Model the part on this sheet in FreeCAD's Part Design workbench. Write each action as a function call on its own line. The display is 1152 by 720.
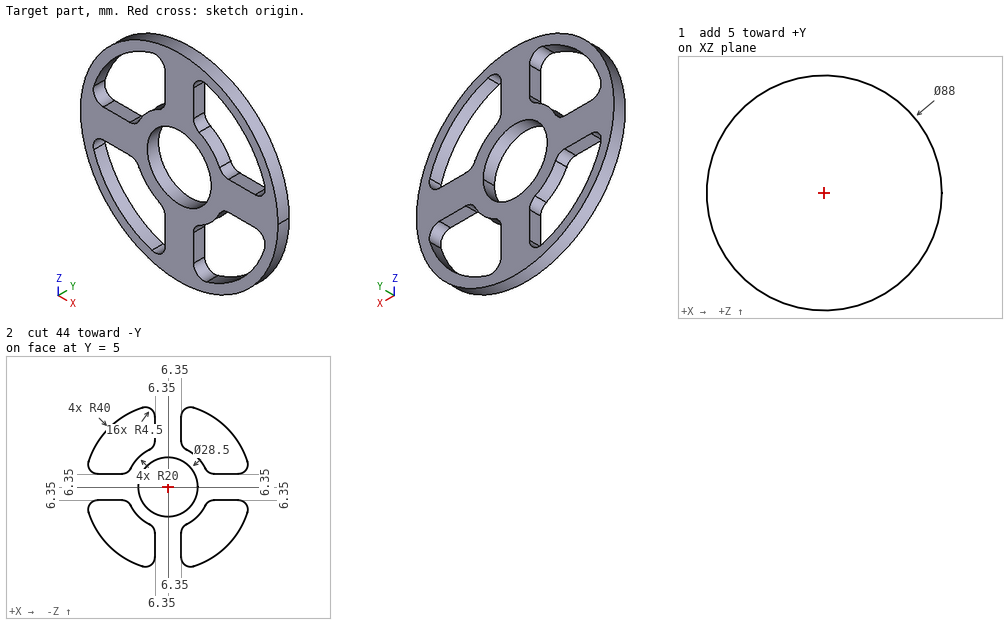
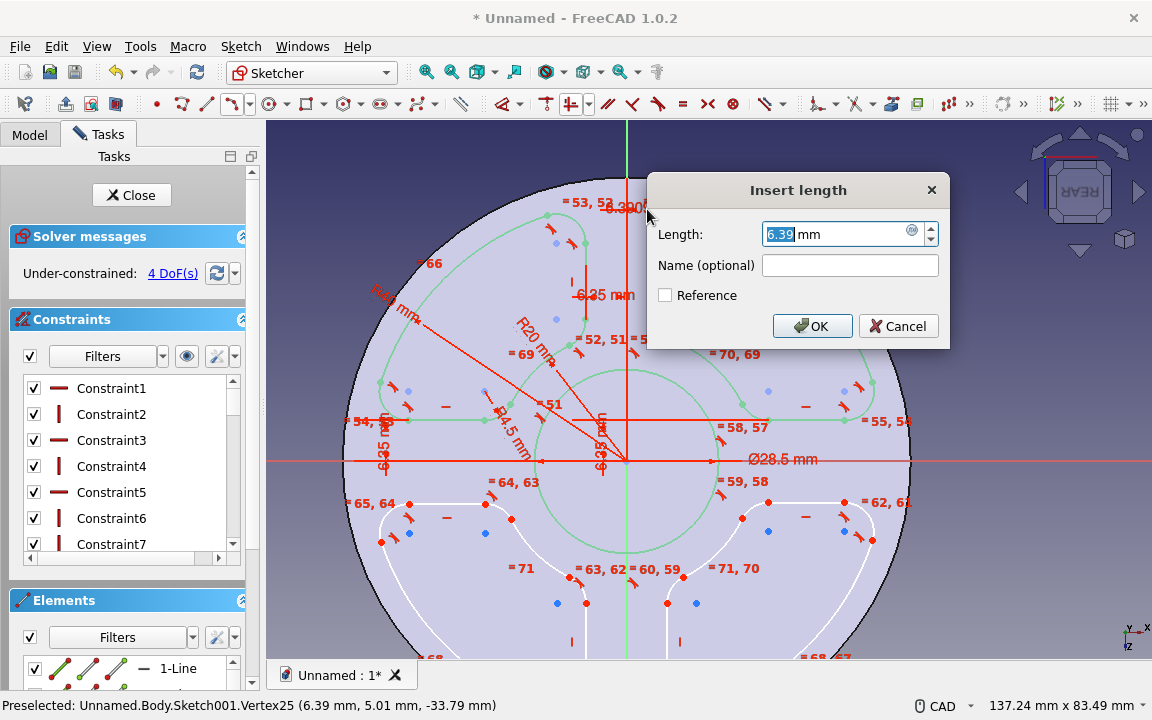
text(6.35)
key(Return)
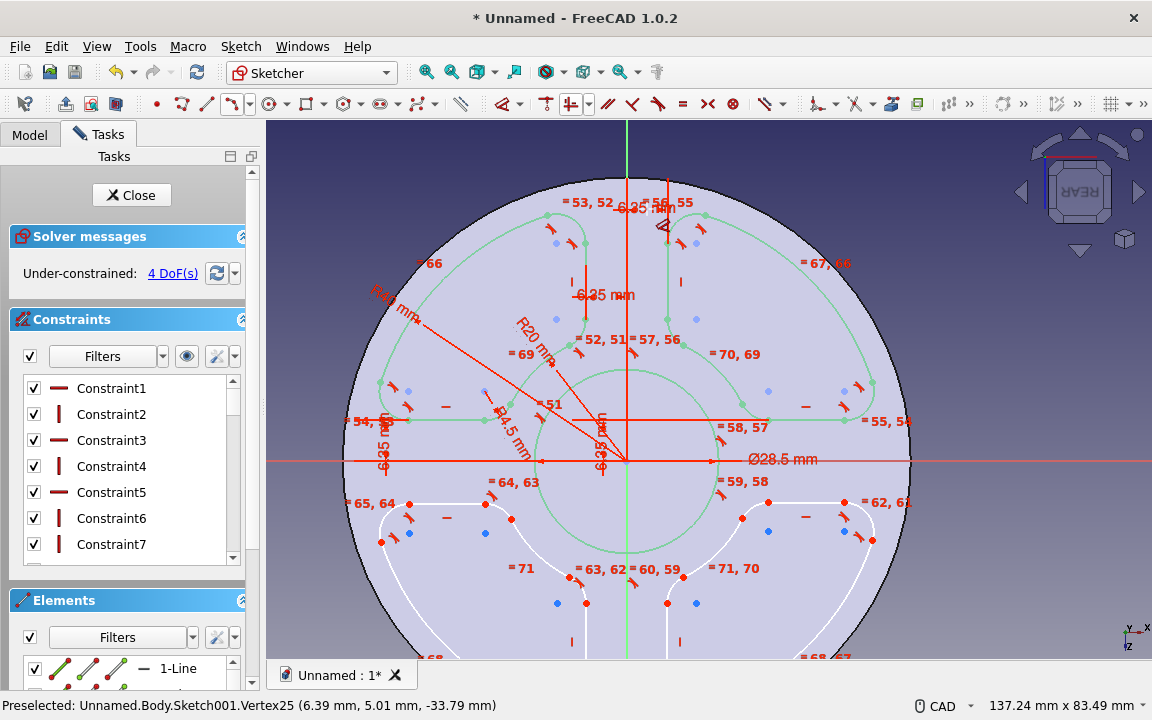
click(845, 503)
click(879, 482)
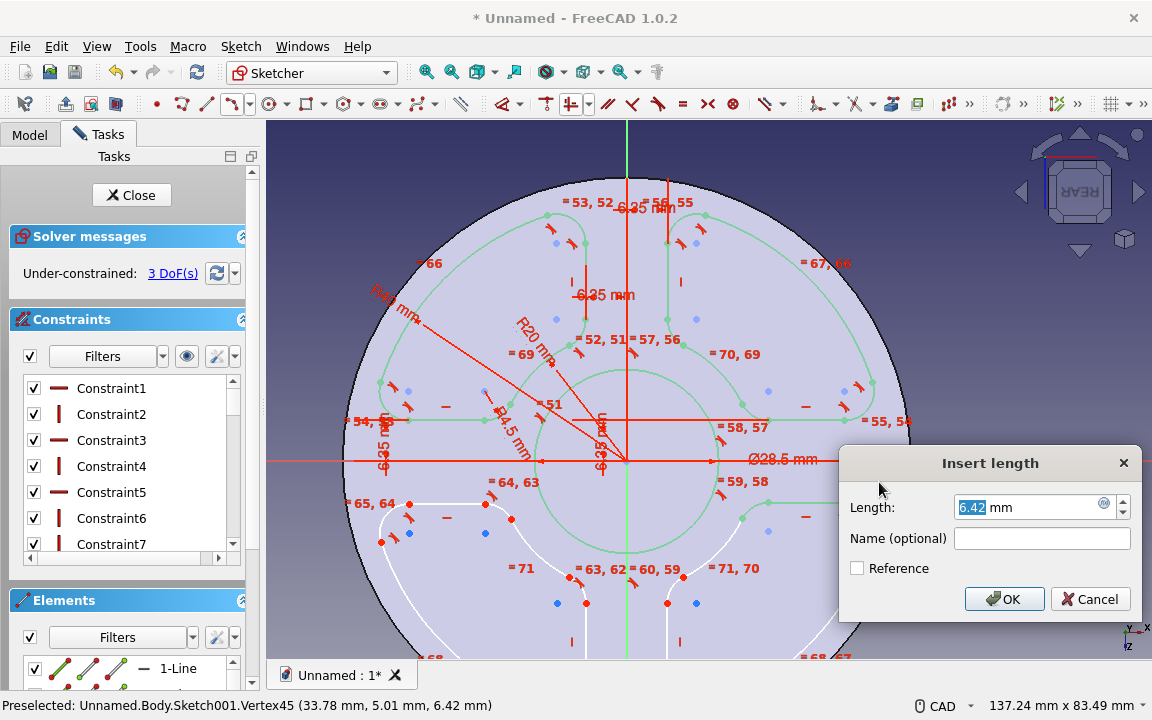
text(6.35)
key(Return)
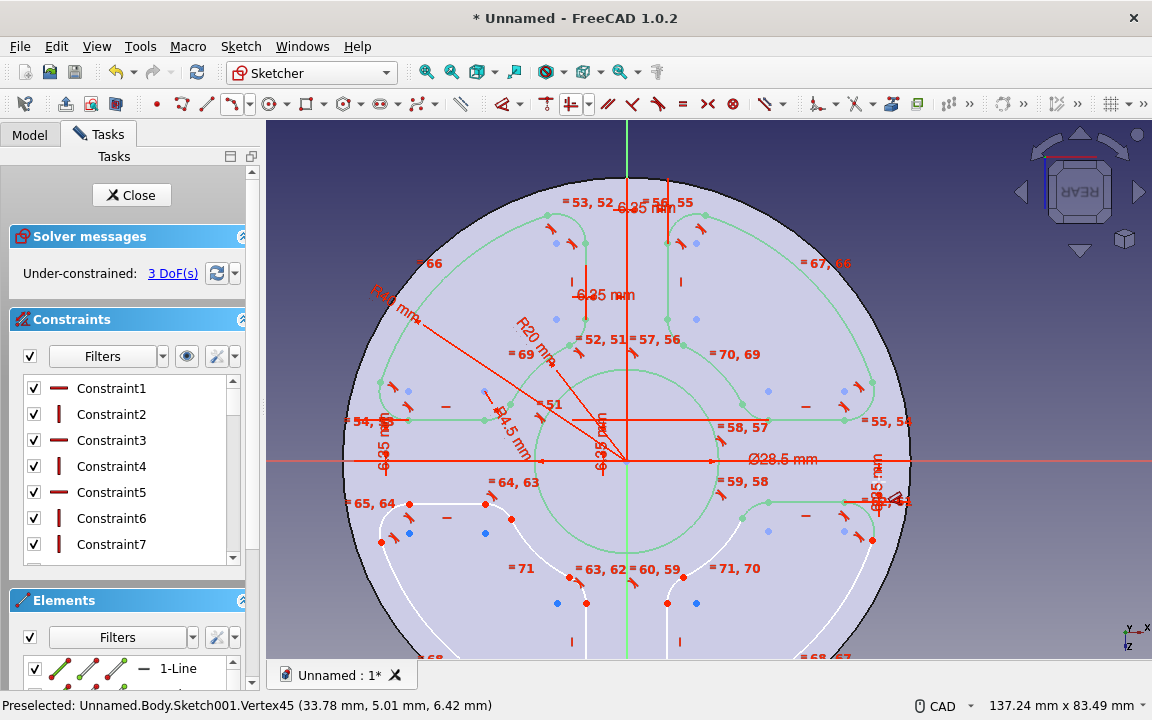
click(667, 604)
click(647, 403)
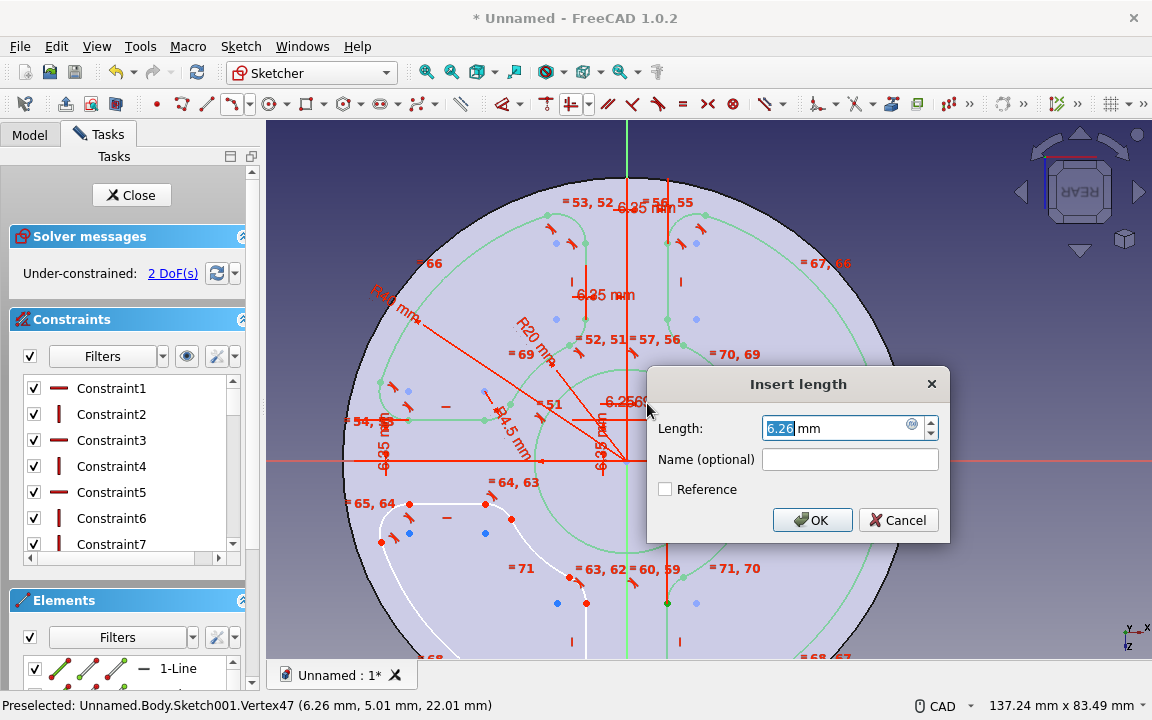
text(6.35)
key(Return)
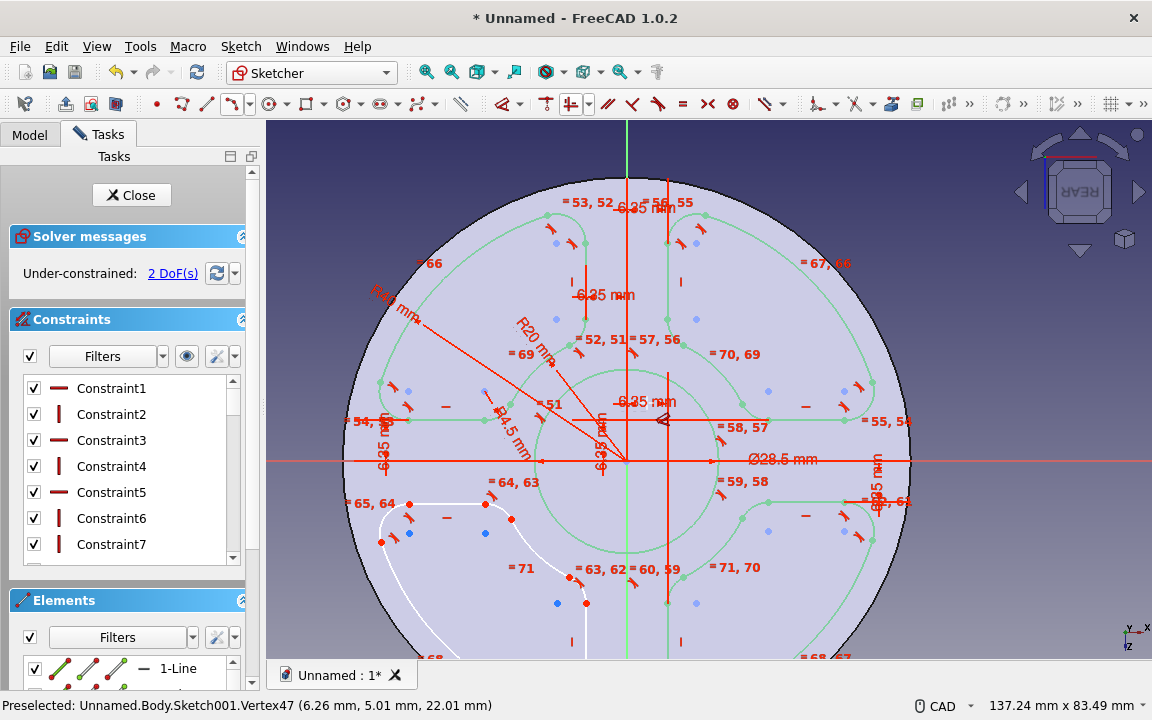
scroll(669, 243, down, 2)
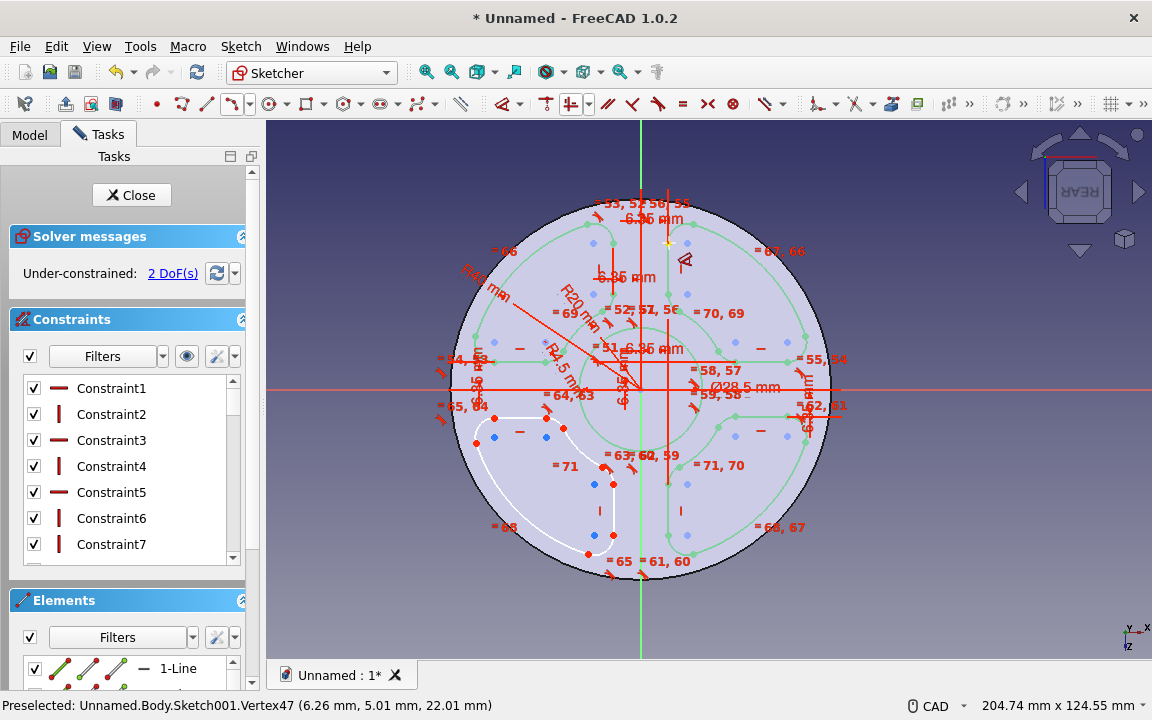
scroll(614, 536, up, 2)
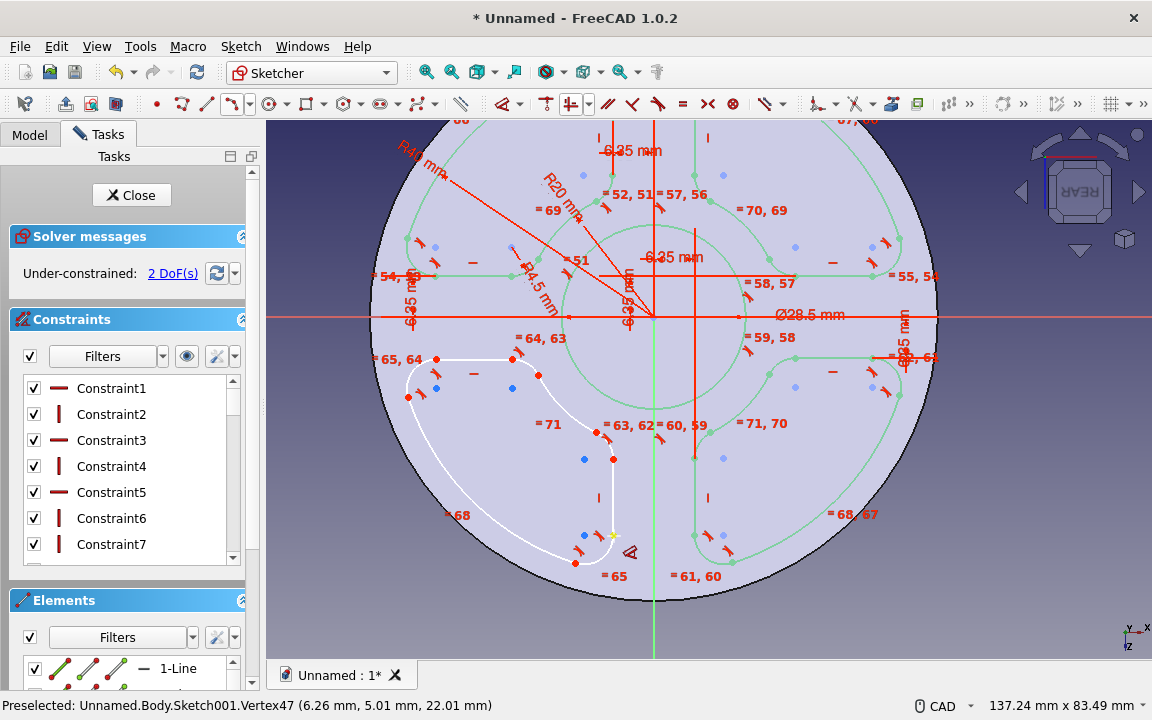
click(613, 535)
click(633, 569)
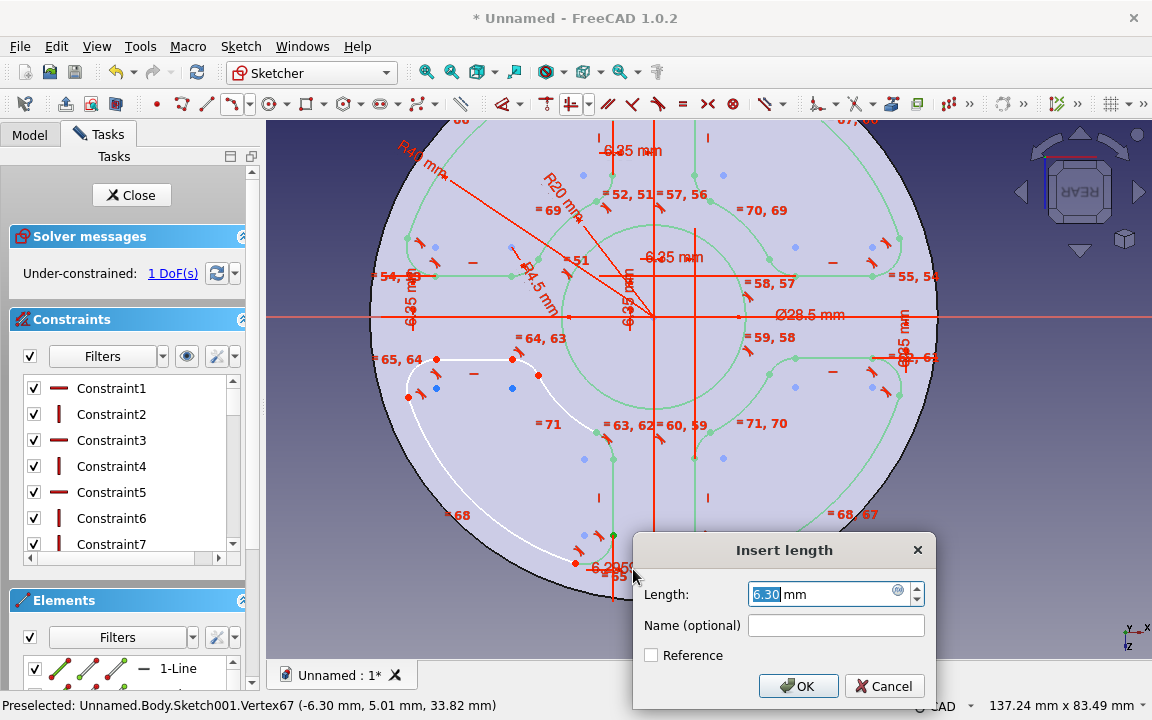
text(6.35)
key(Return)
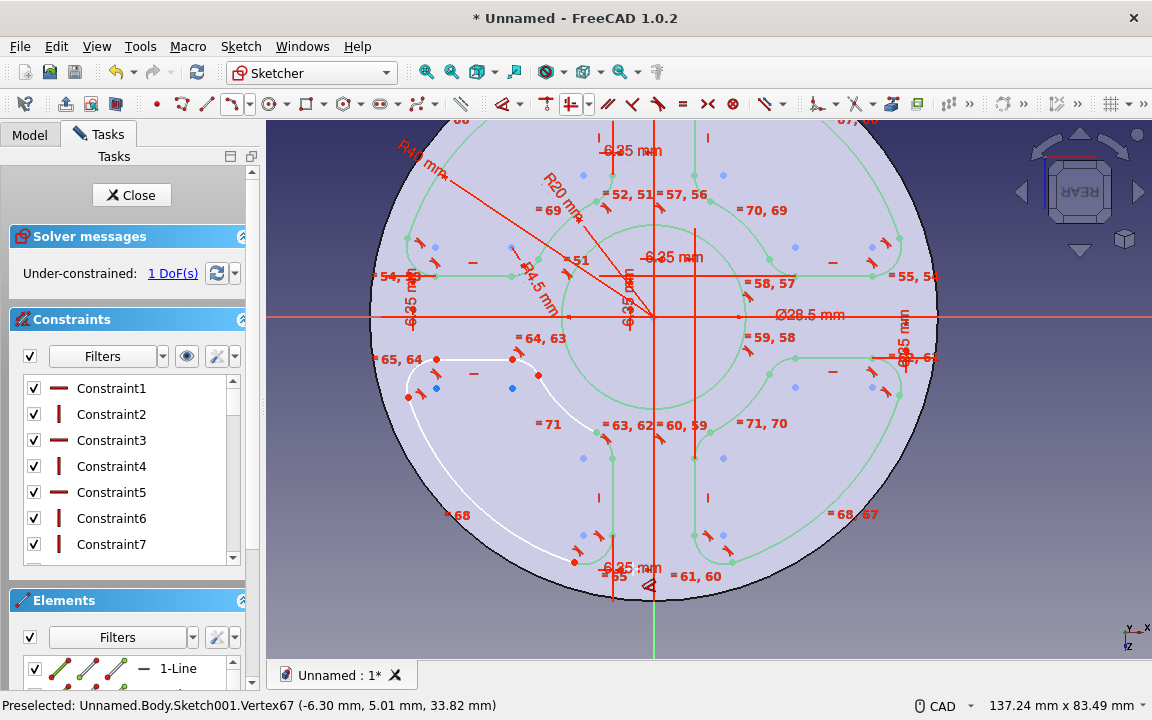
click(513, 360)
click(479, 338)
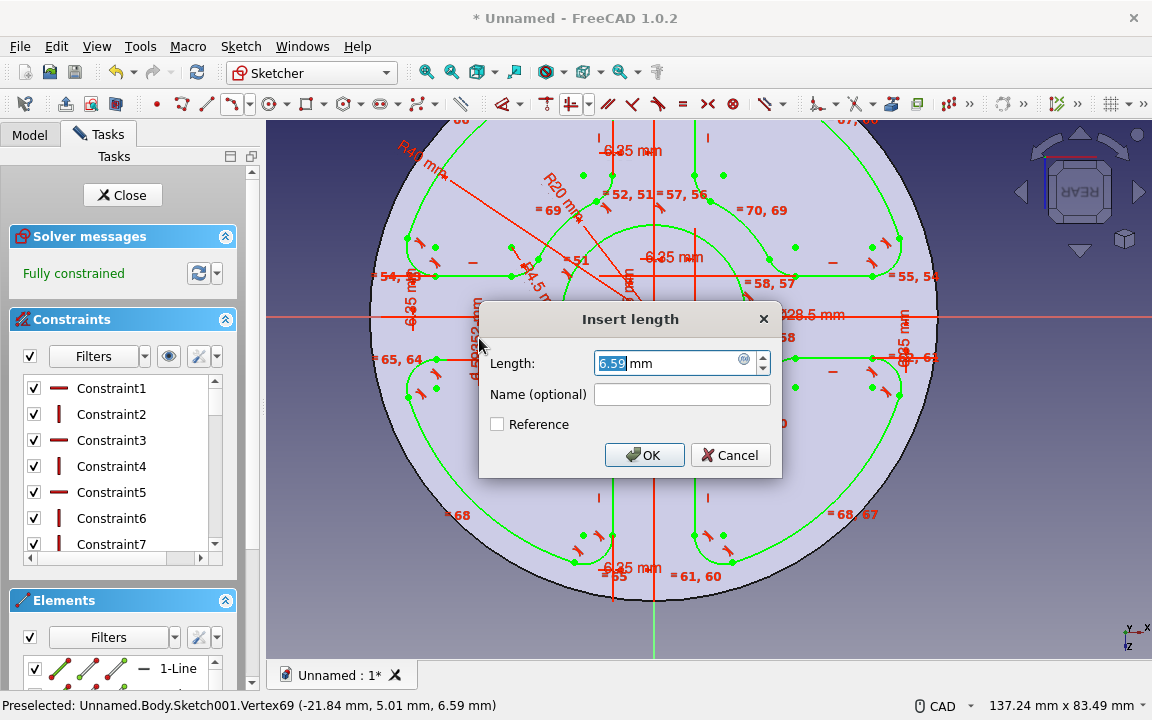
text(6.35)
key(Return)
key(Escape)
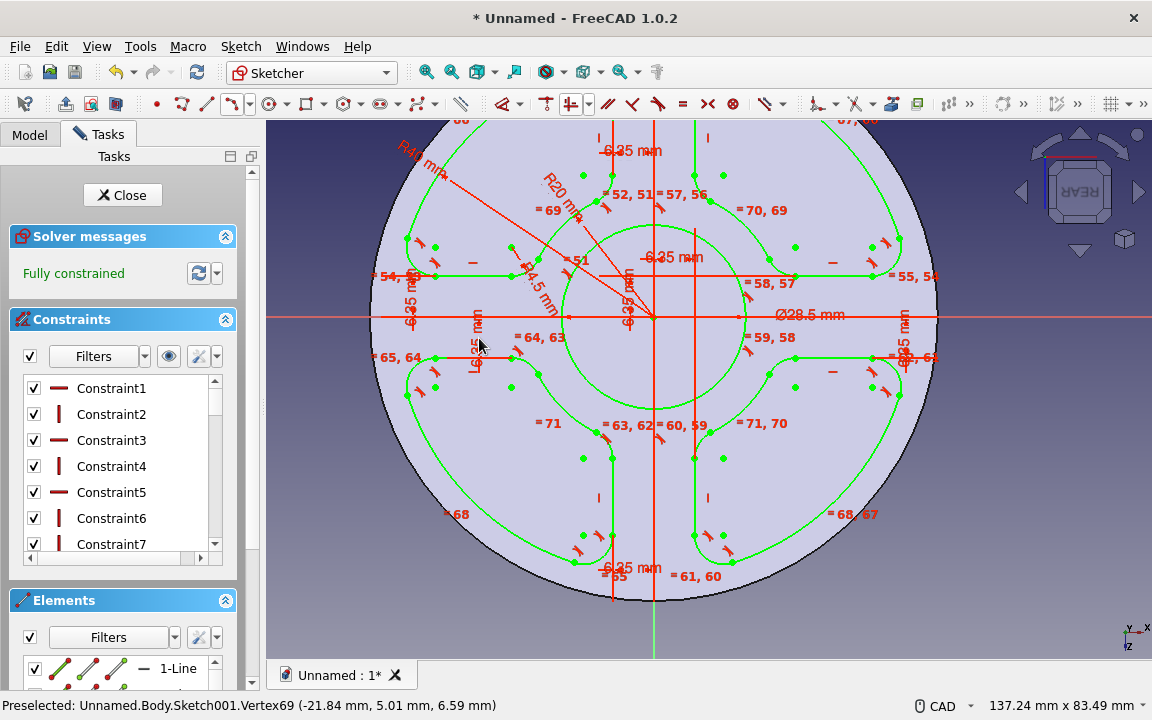
click(123, 195)